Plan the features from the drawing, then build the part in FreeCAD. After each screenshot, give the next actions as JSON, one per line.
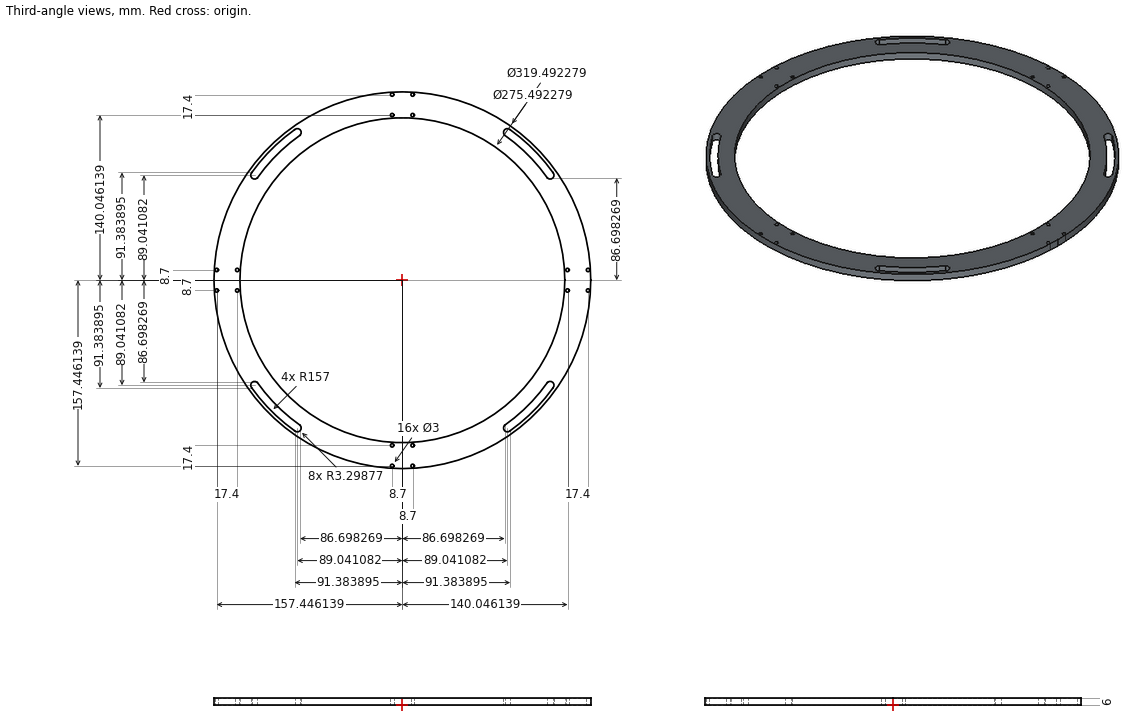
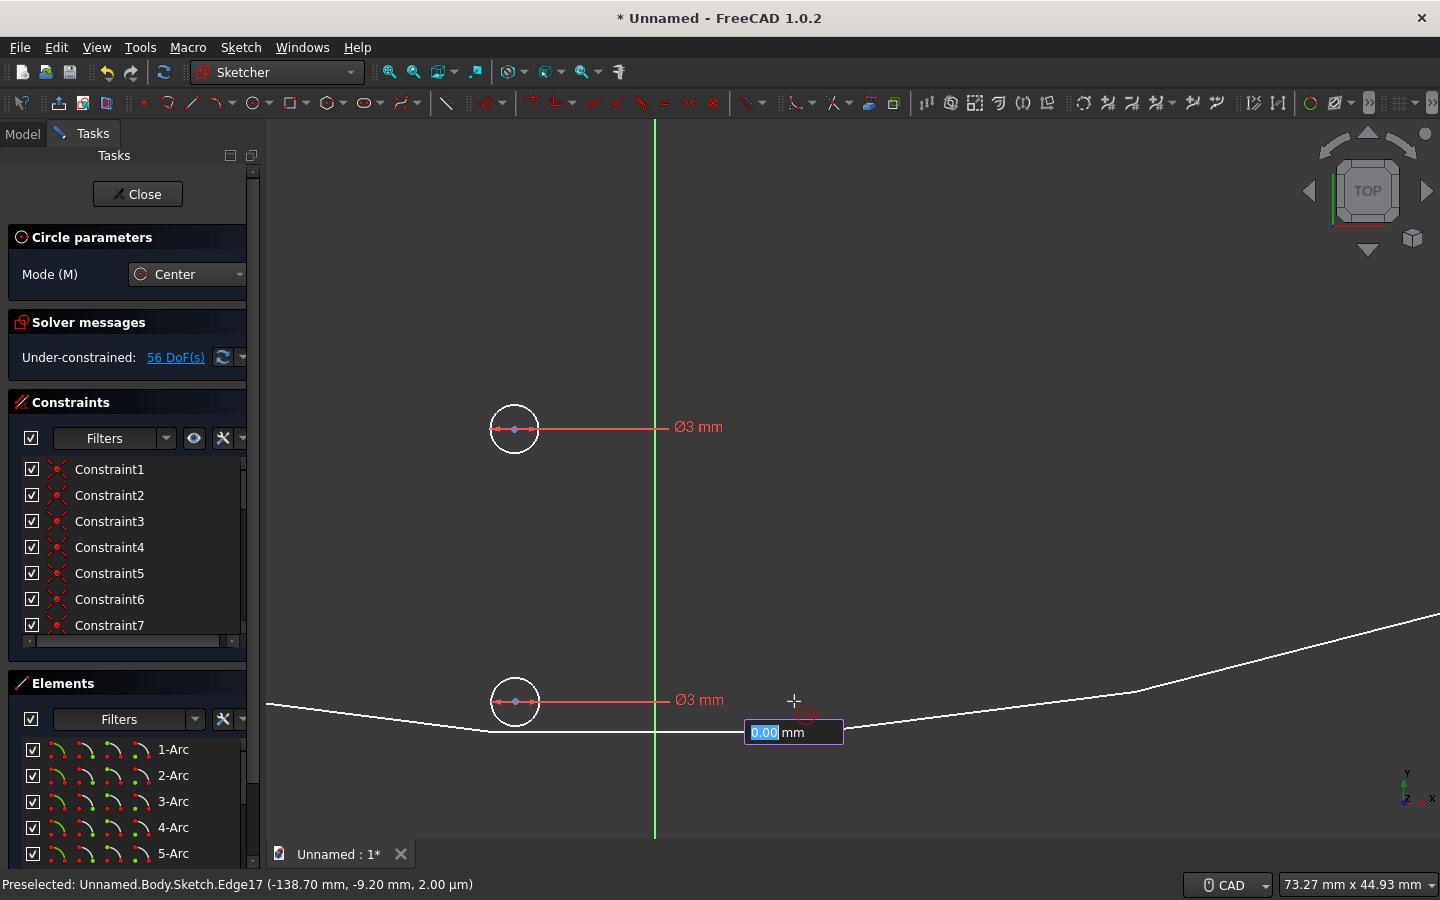
{"action": "scroll", "coordinate": [797, 709], "scroll_direction": "down", "scroll_amount": 12}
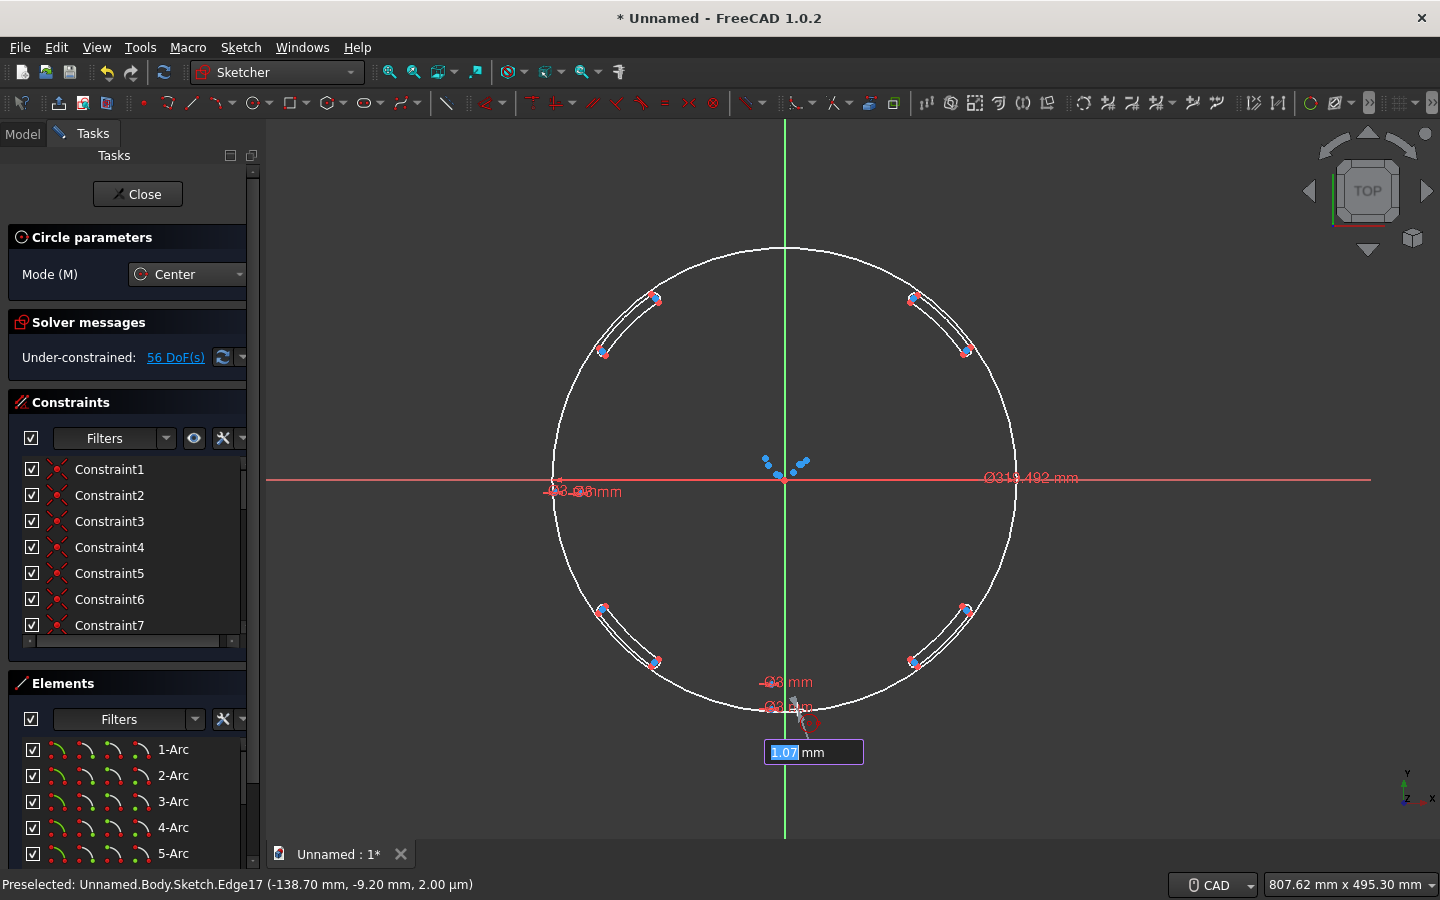
{"action": "scroll", "coordinate": [799, 707], "scroll_direction": "up", "scroll_amount": 7}
{"action": "mouse_move", "coordinate": [797, 706]}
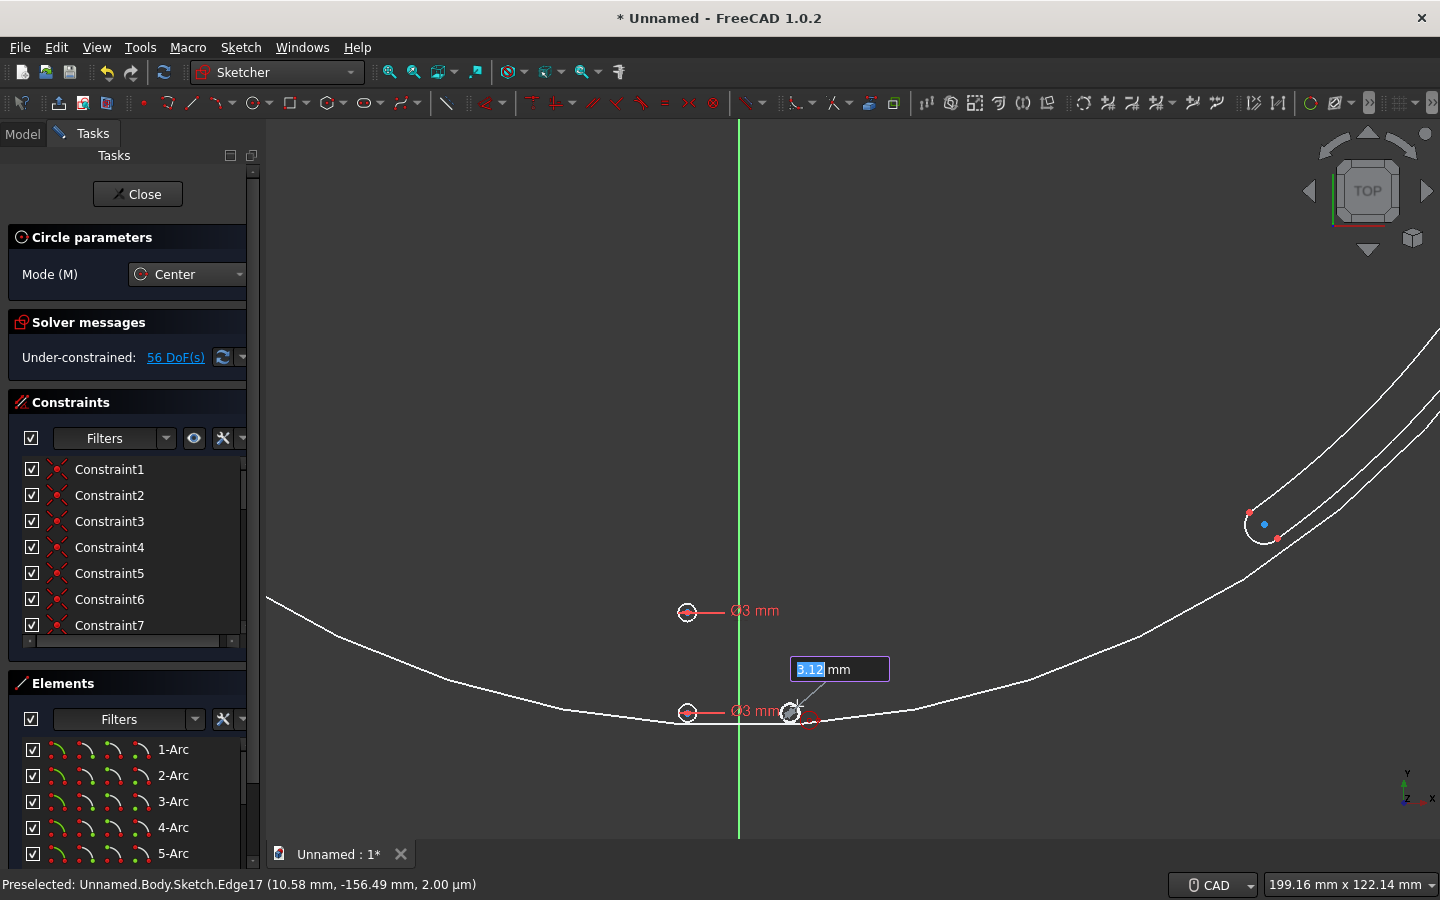
{"action": "type", "text": "3"}
{"action": "key", "text": "Return"}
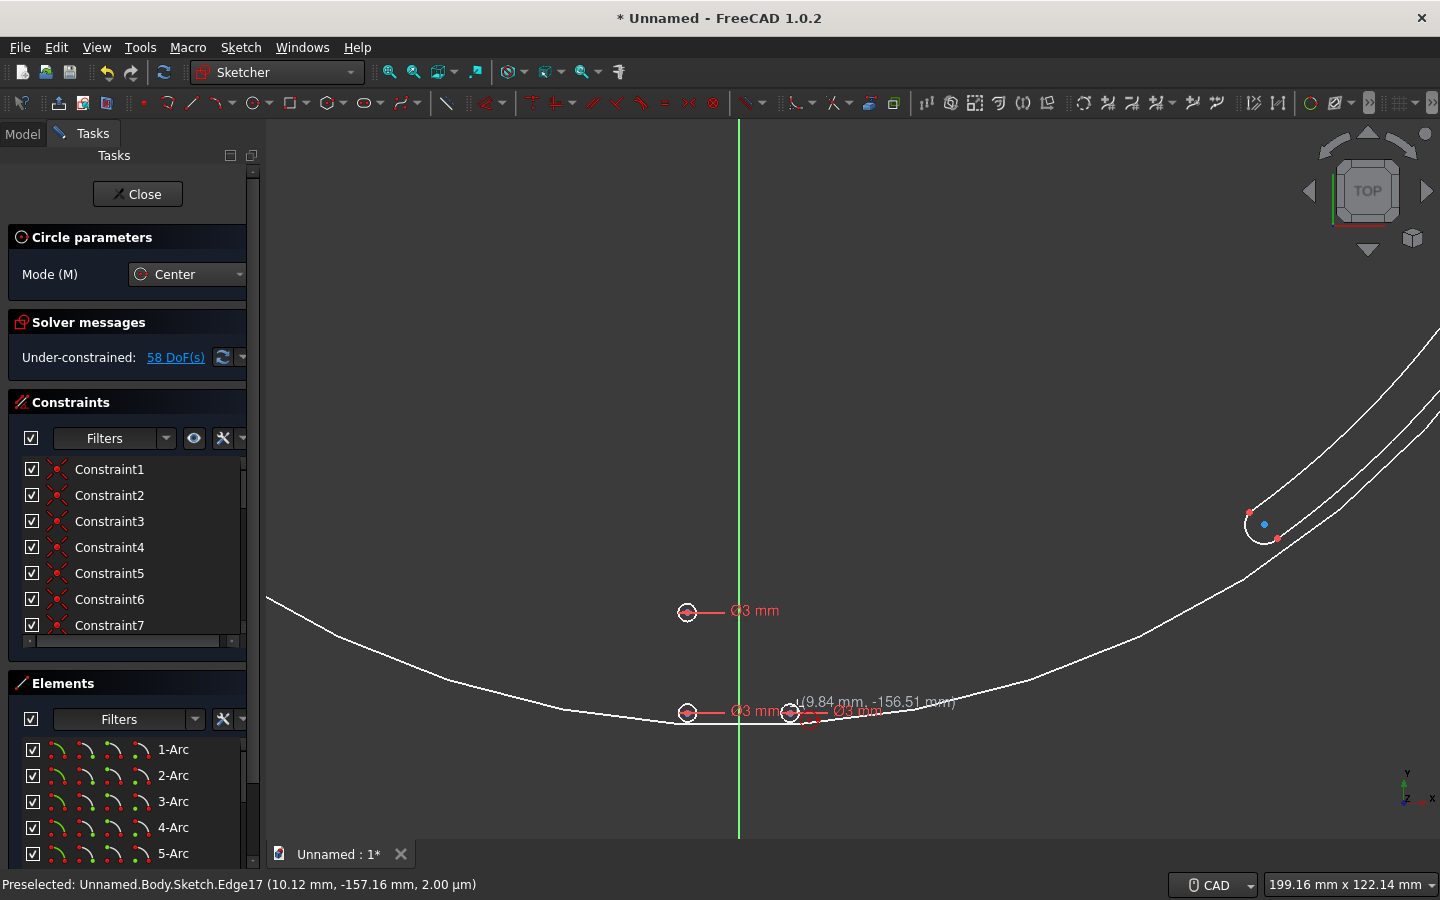
{"action": "scroll", "coordinate": [790, 610], "scroll_direction": "up", "scroll_amount": 5}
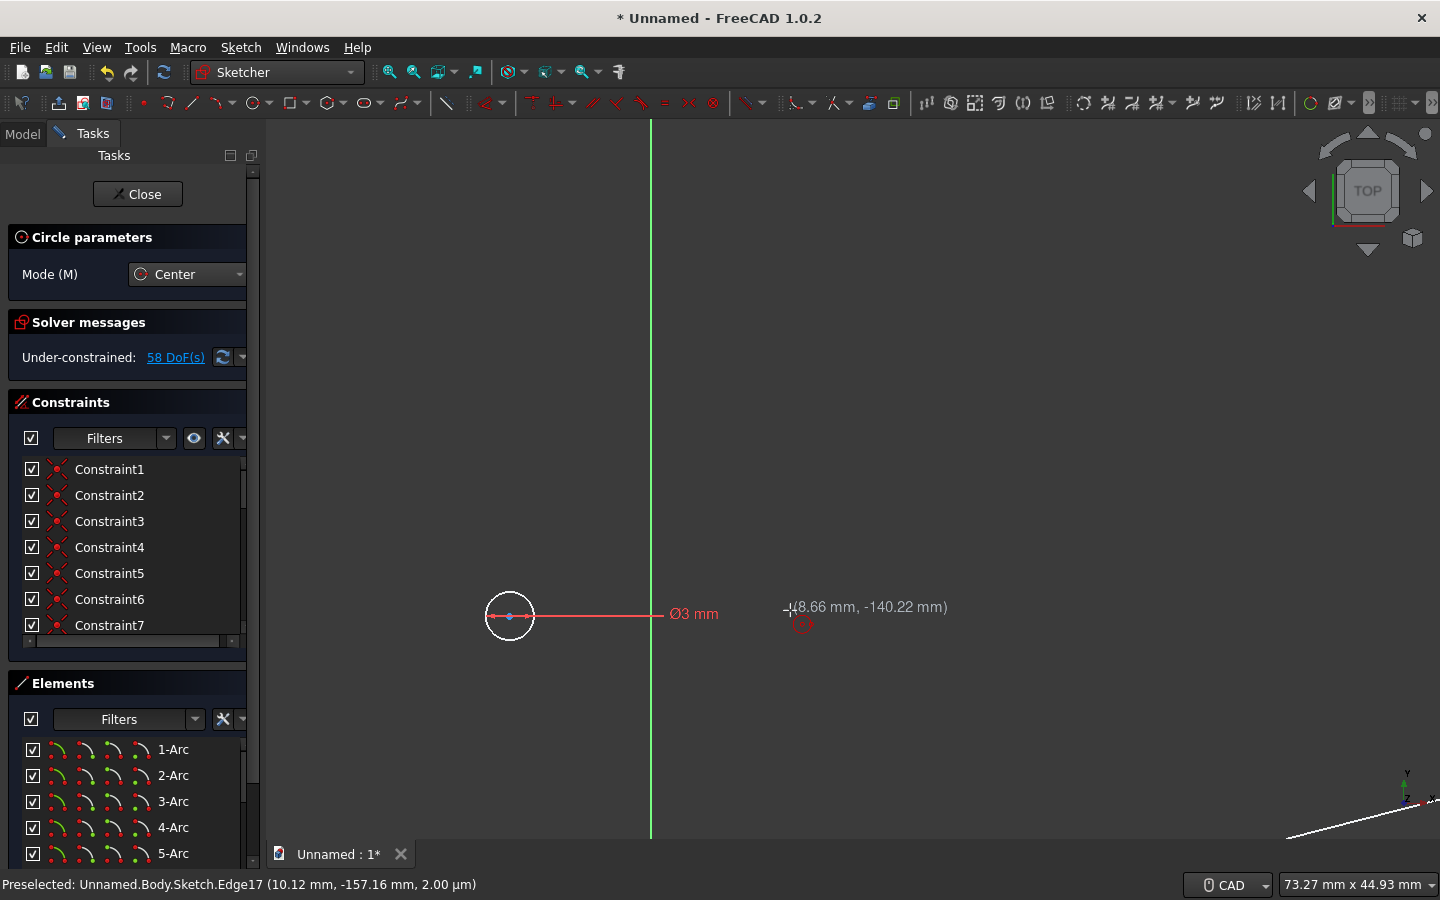
{"action": "scroll", "coordinate": [798, 690], "scroll_direction": "down", "scroll_amount": 12}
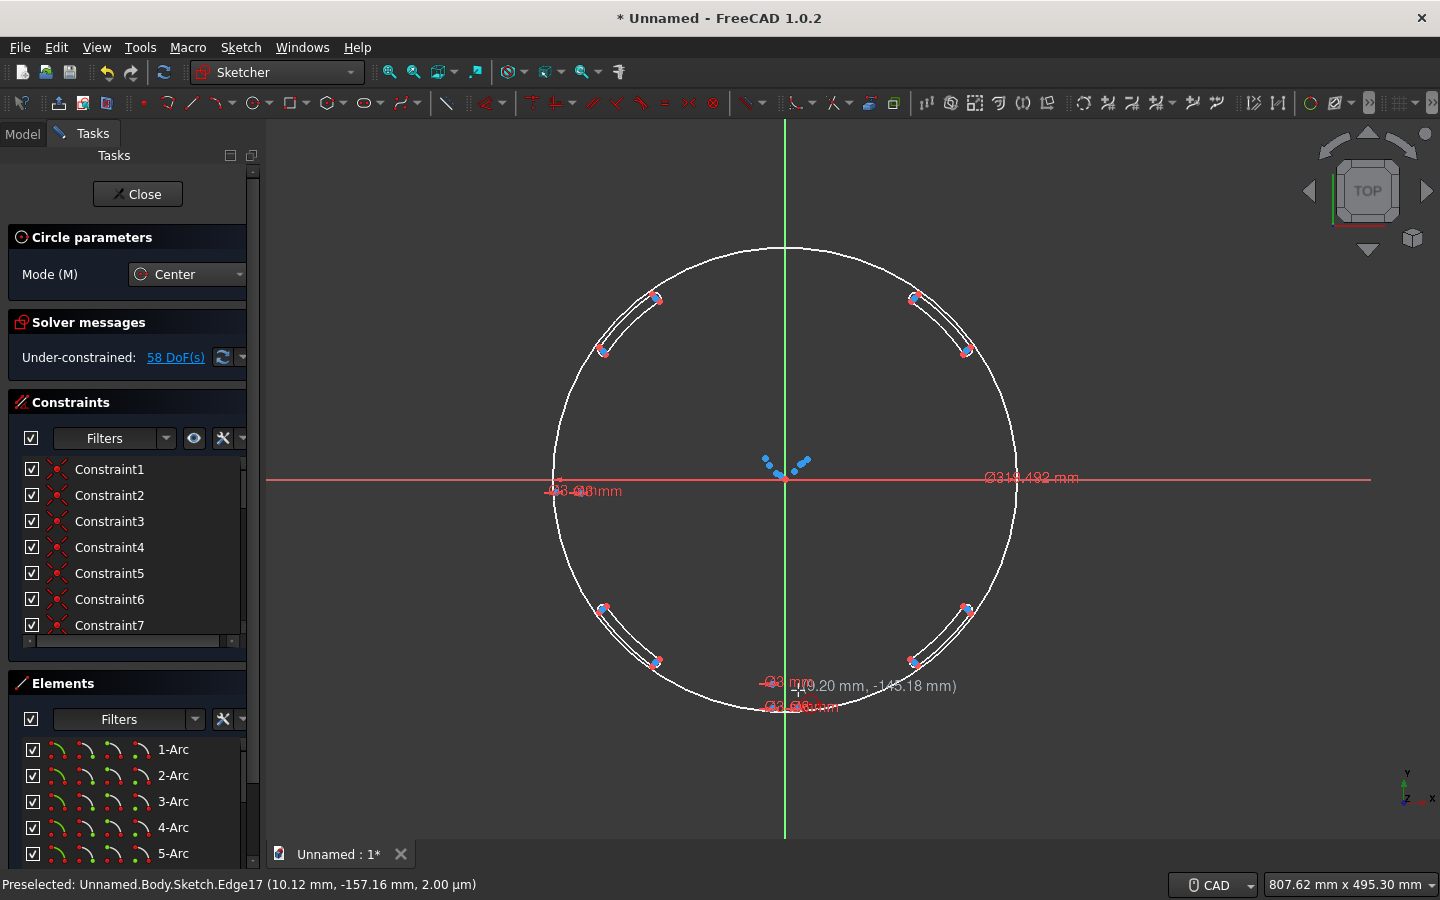
{"action": "scroll", "coordinate": [798, 683], "scroll_direction": "up", "scroll_amount": 2}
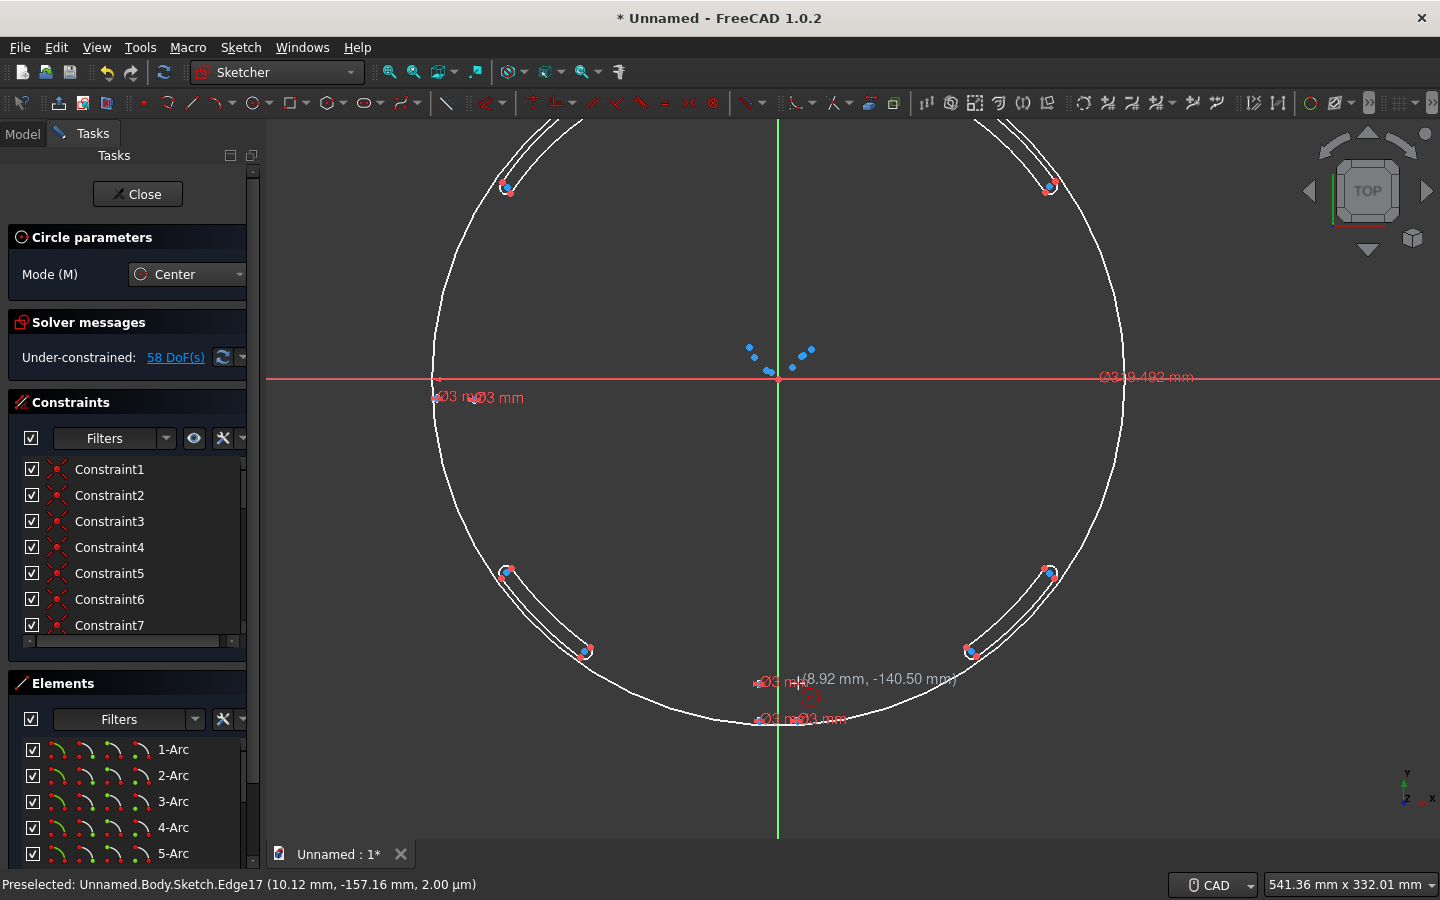
{"action": "left_click", "coordinate": [797, 683]}
{"action": "mouse_move", "coordinate": [800, 681]}